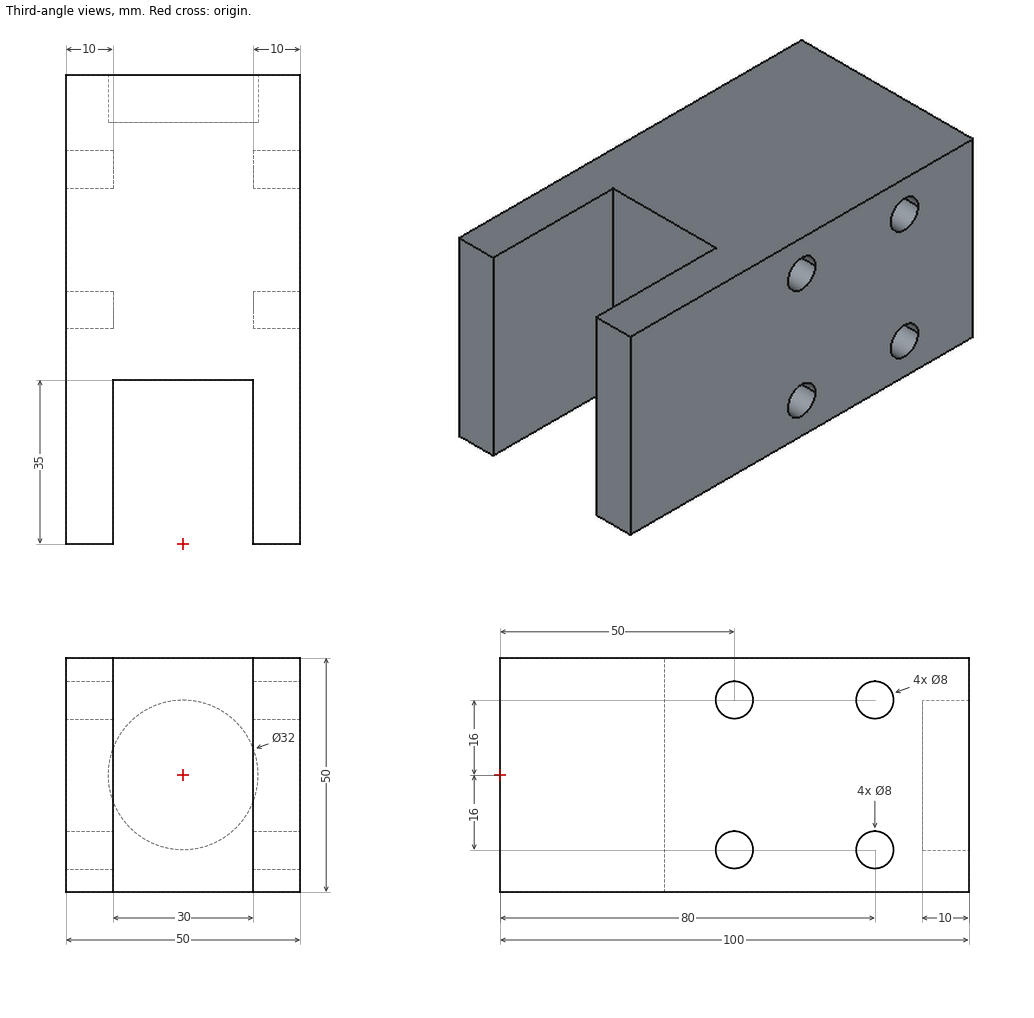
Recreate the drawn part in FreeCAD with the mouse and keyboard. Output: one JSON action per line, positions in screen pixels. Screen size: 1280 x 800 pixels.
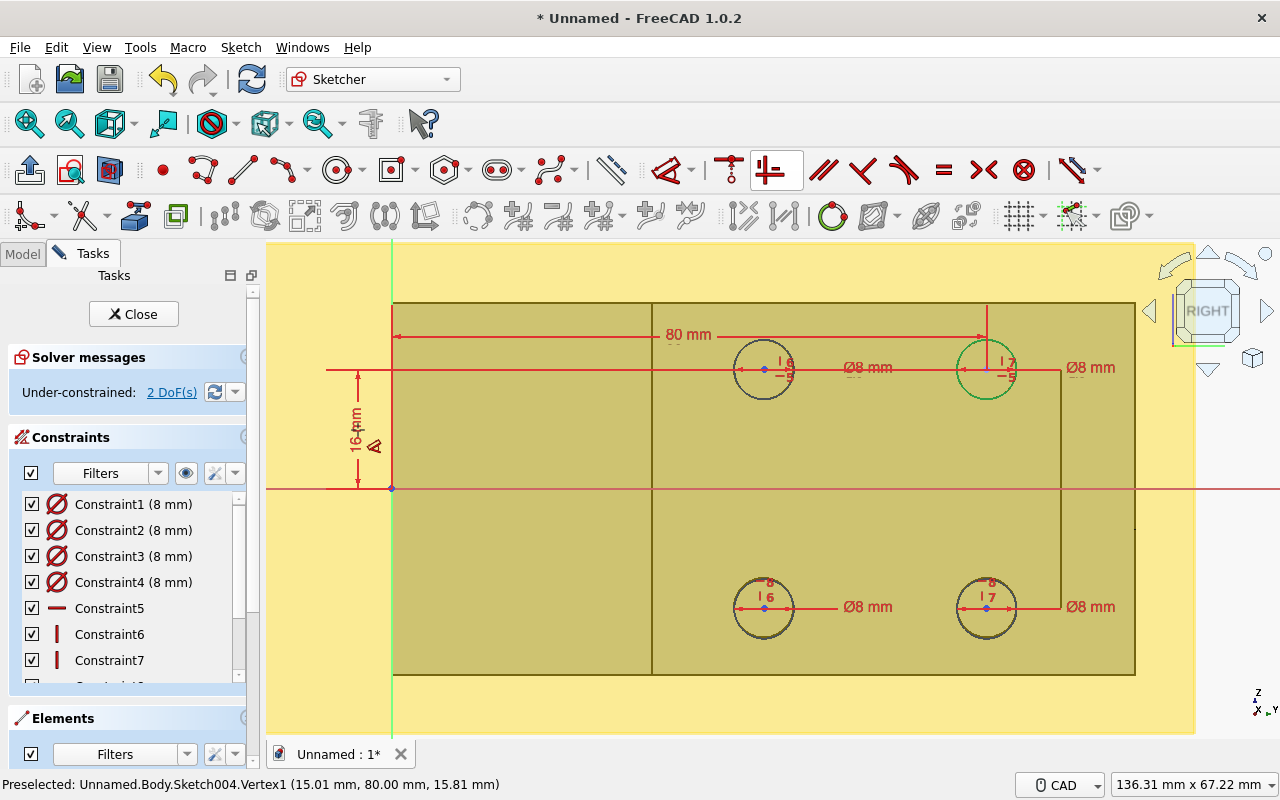
{"action": "left_click", "coordinate": [764, 370]}
{"action": "left_click", "coordinate": [578, 336]}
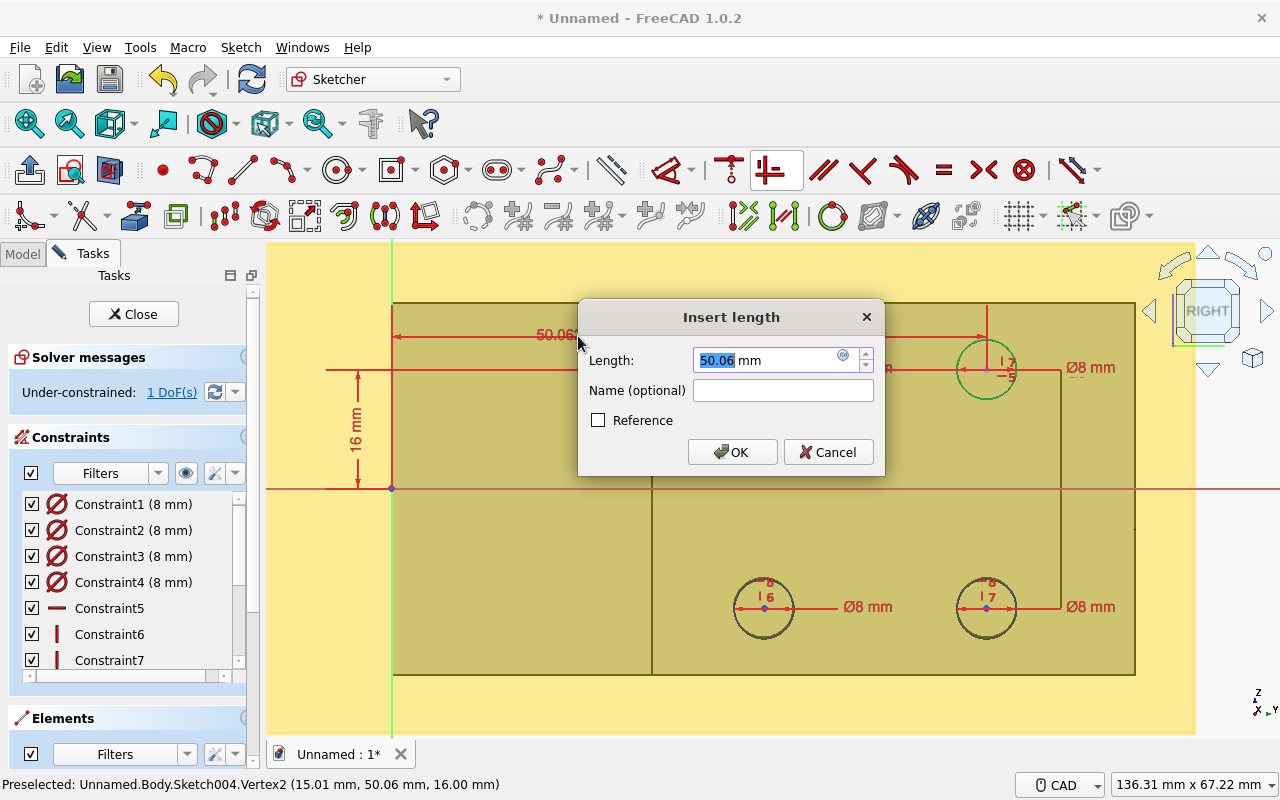
{"action": "type", "text": "50"}
{"action": "key", "text": "Return"}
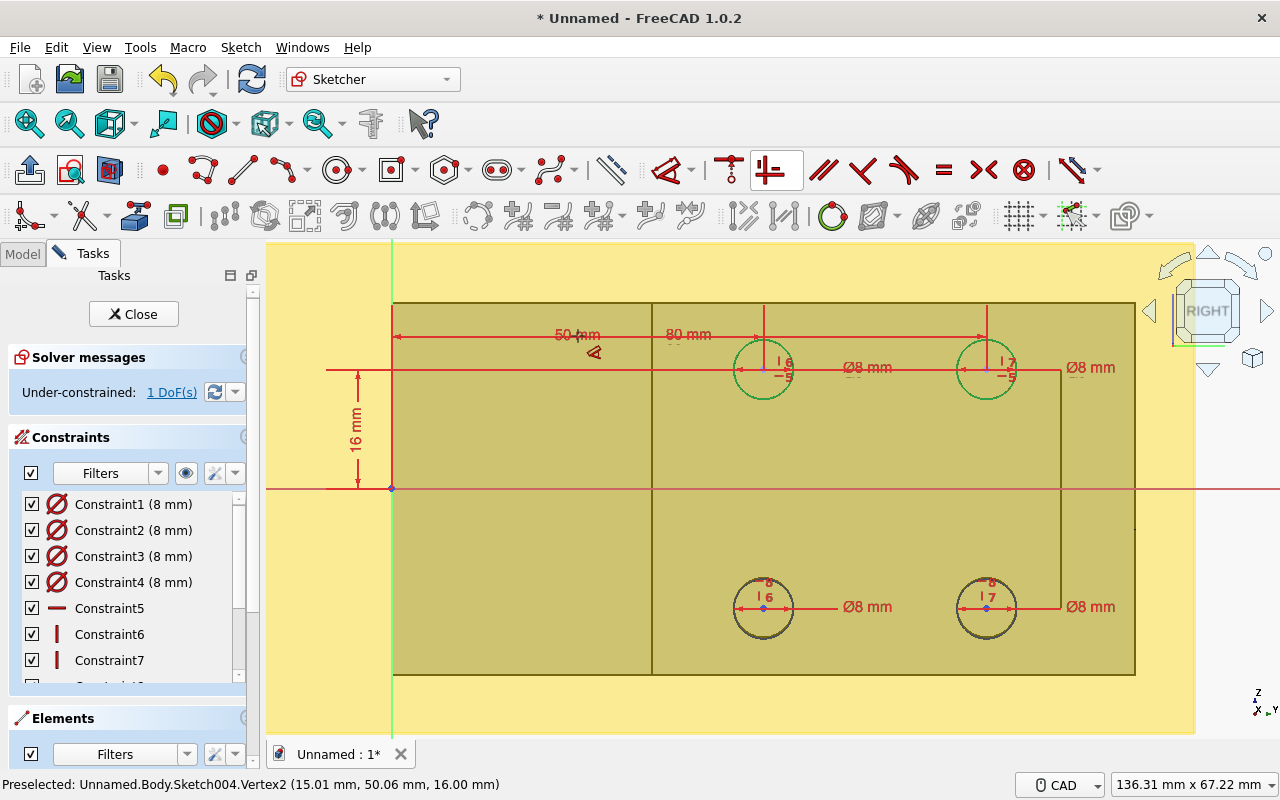
{"action": "left_click", "coordinate": [764, 609]}
{"action": "left_click", "coordinate": [358, 549]}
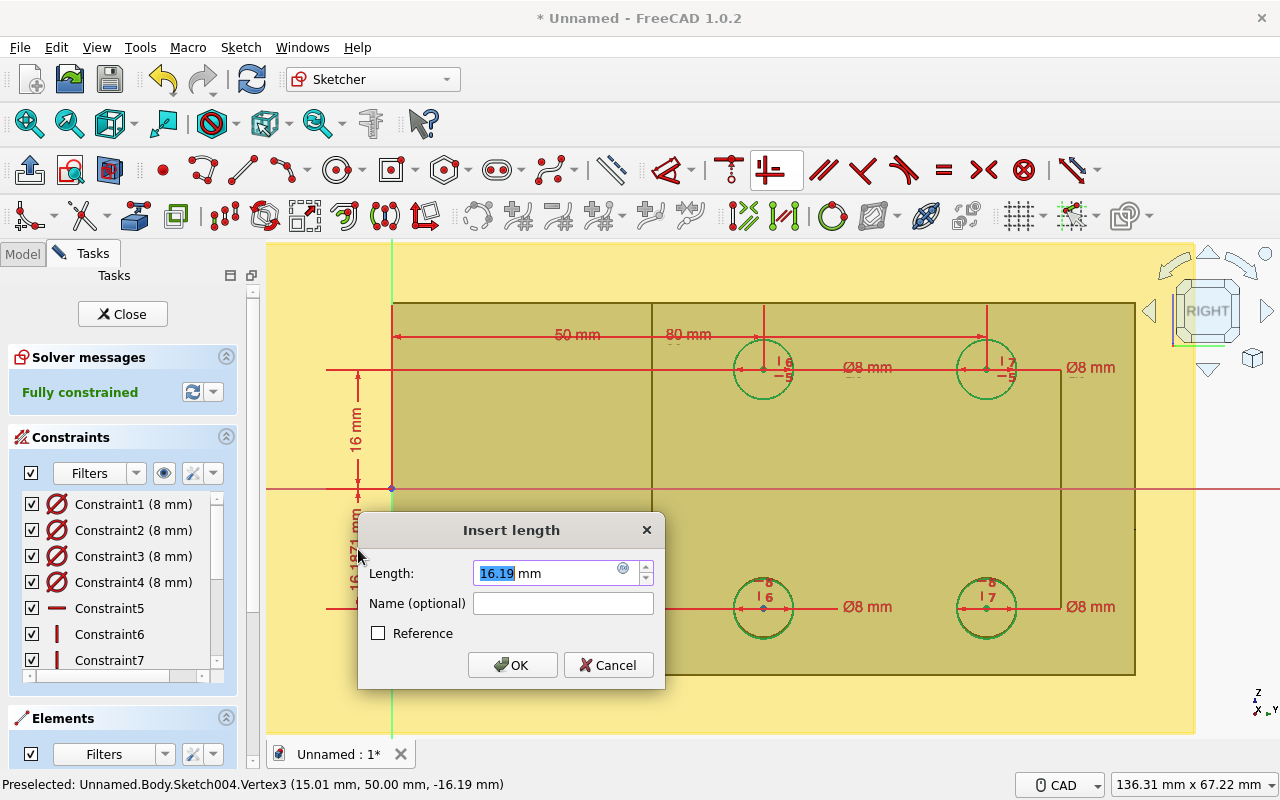
{"action": "type", "text": "16"}
{"action": "key", "text": "Return"}
{"action": "key", "text": "Escape"}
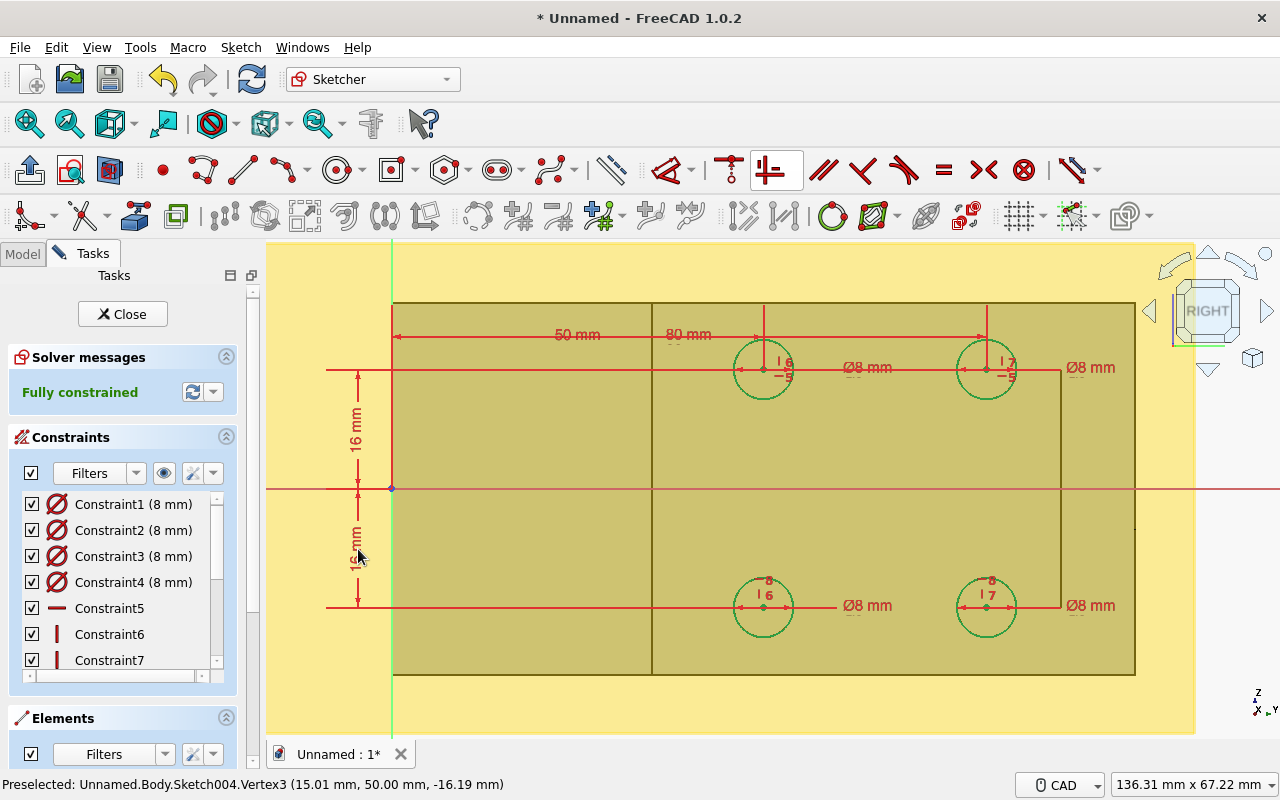
{"action": "left_click", "coordinate": [123, 314]}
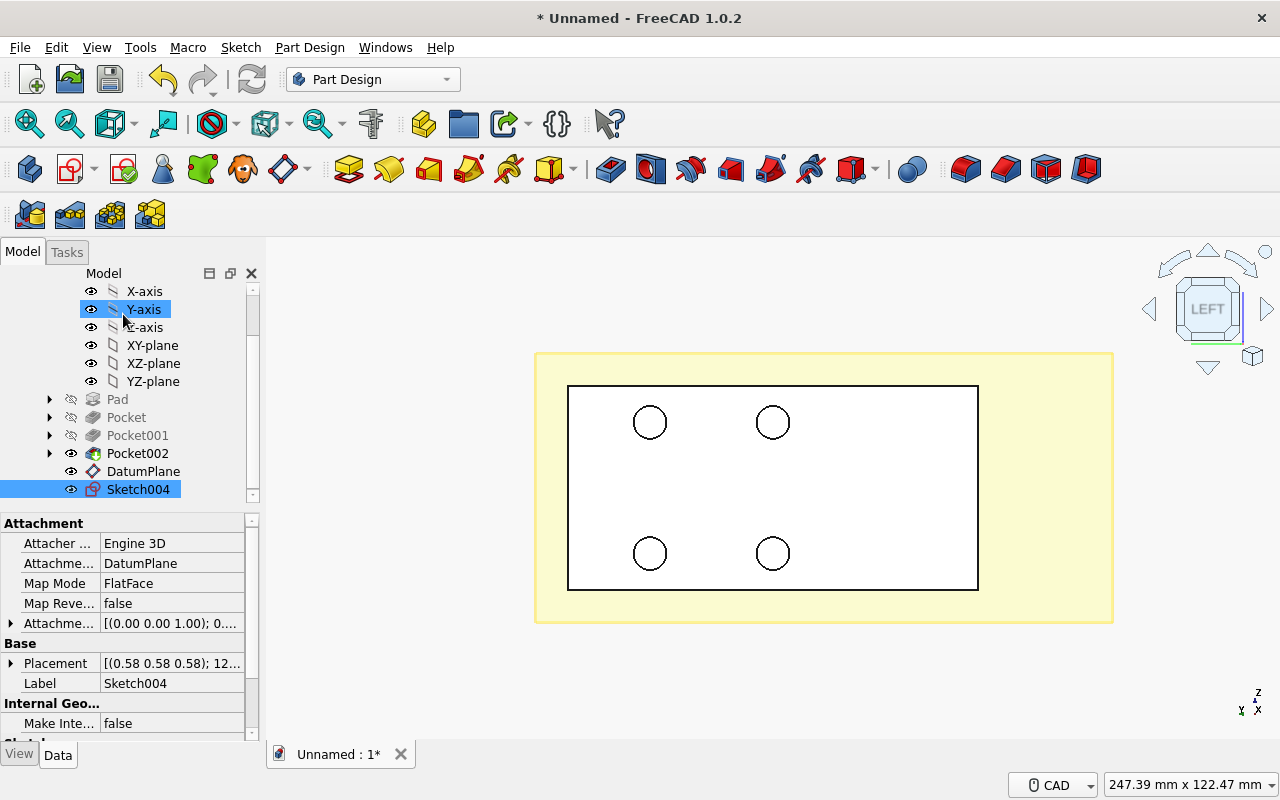
{"action": "left_click", "coordinate": [612, 170]}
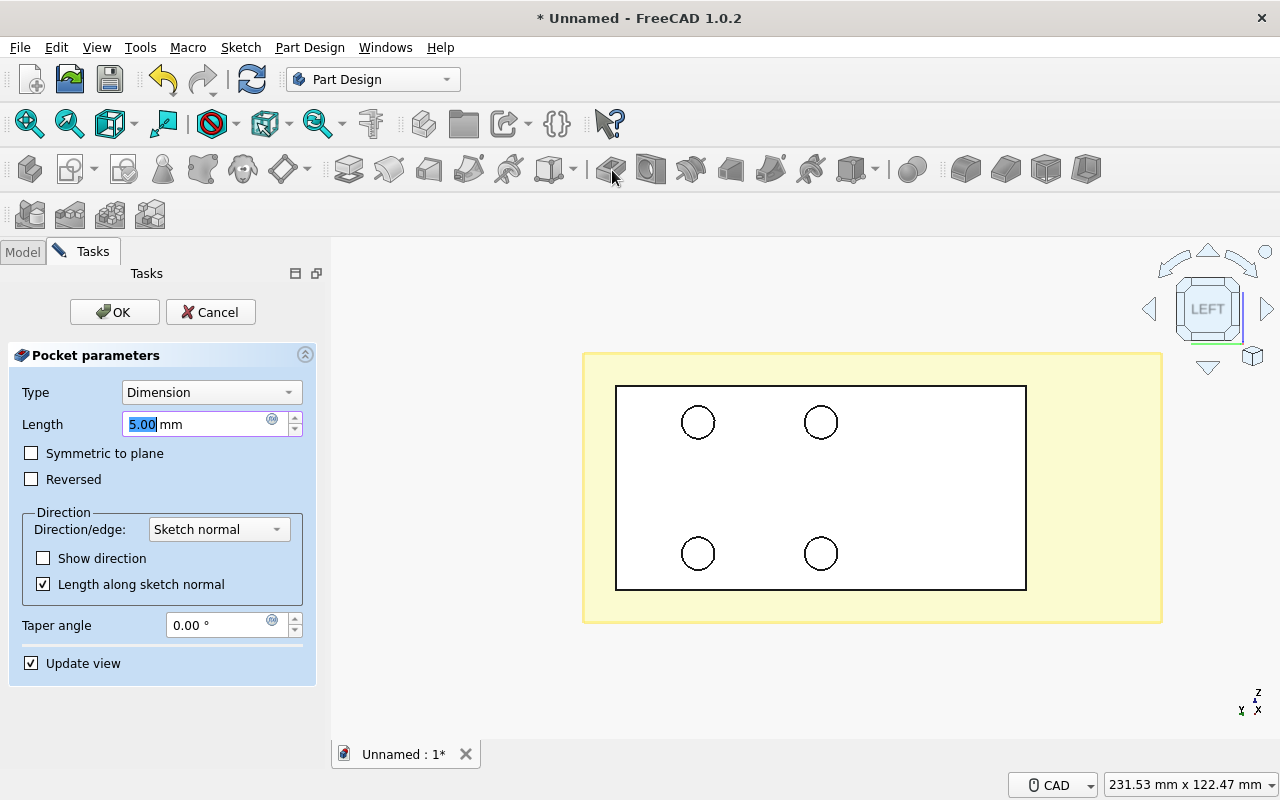
{"action": "type", "text": "10"}
{"action": "key", "text": "Tab"}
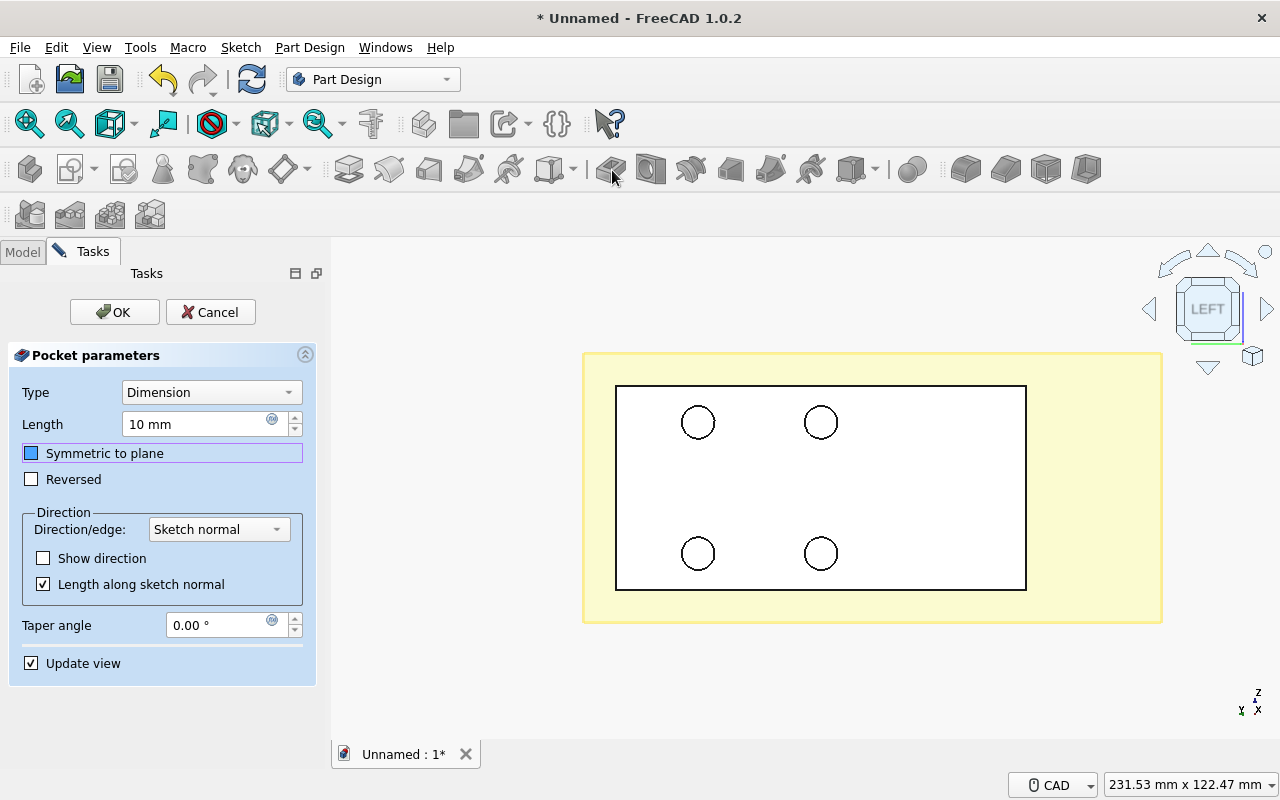
{"action": "left_click", "coordinate": [30, 479]}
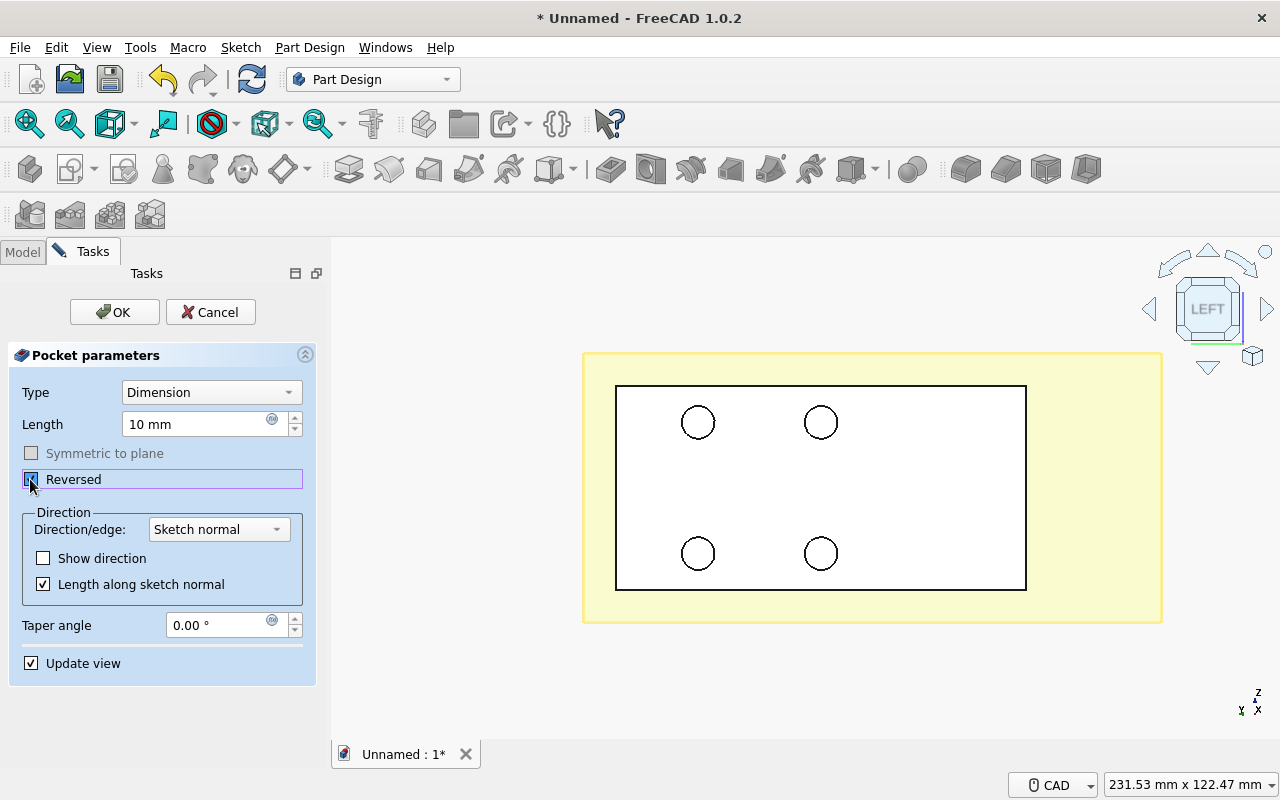
{"action": "left_click", "coordinate": [115, 312]}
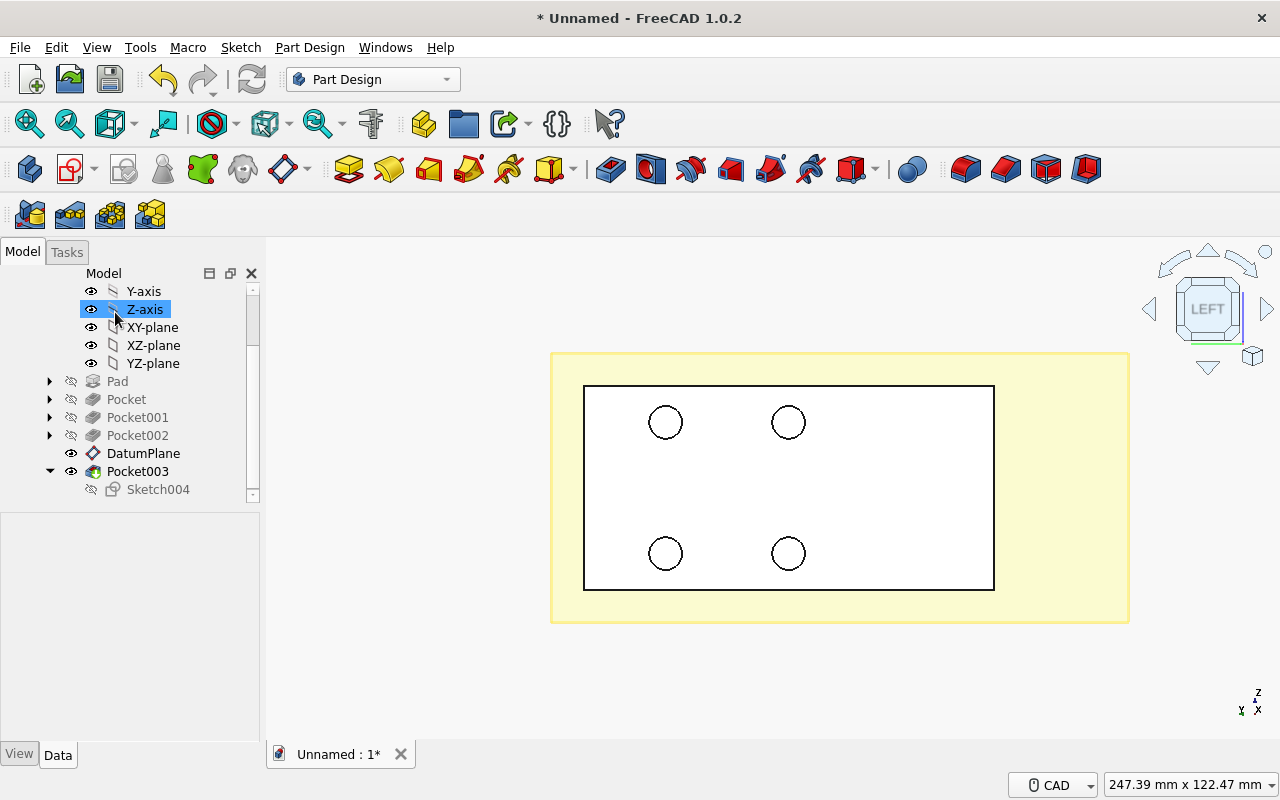
{"action": "left_click", "coordinate": [116, 453]}
{"action": "key", "text": "space"}